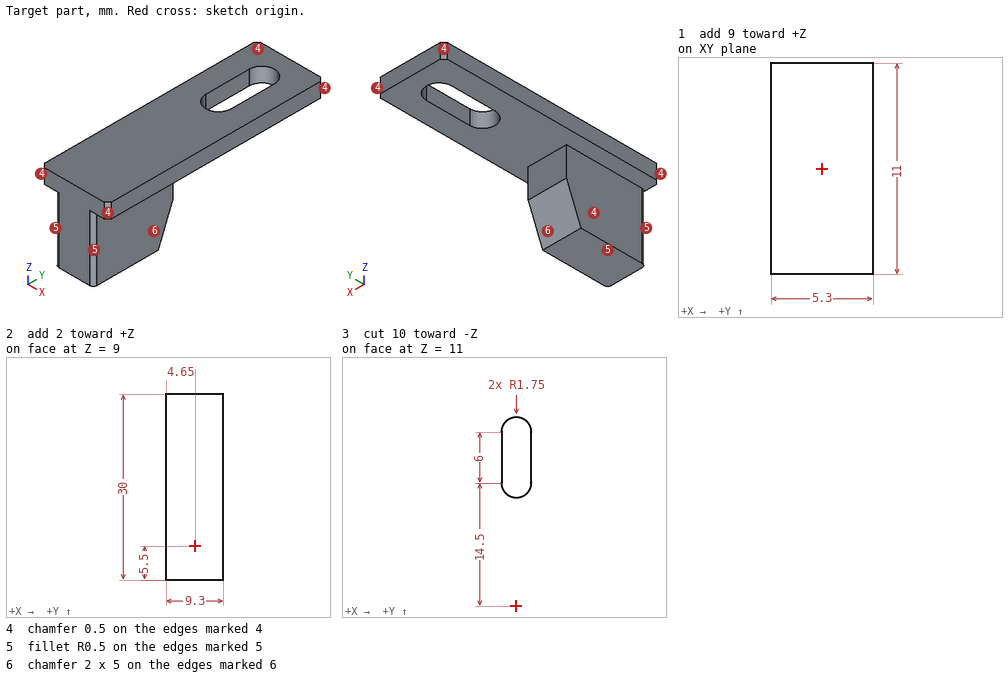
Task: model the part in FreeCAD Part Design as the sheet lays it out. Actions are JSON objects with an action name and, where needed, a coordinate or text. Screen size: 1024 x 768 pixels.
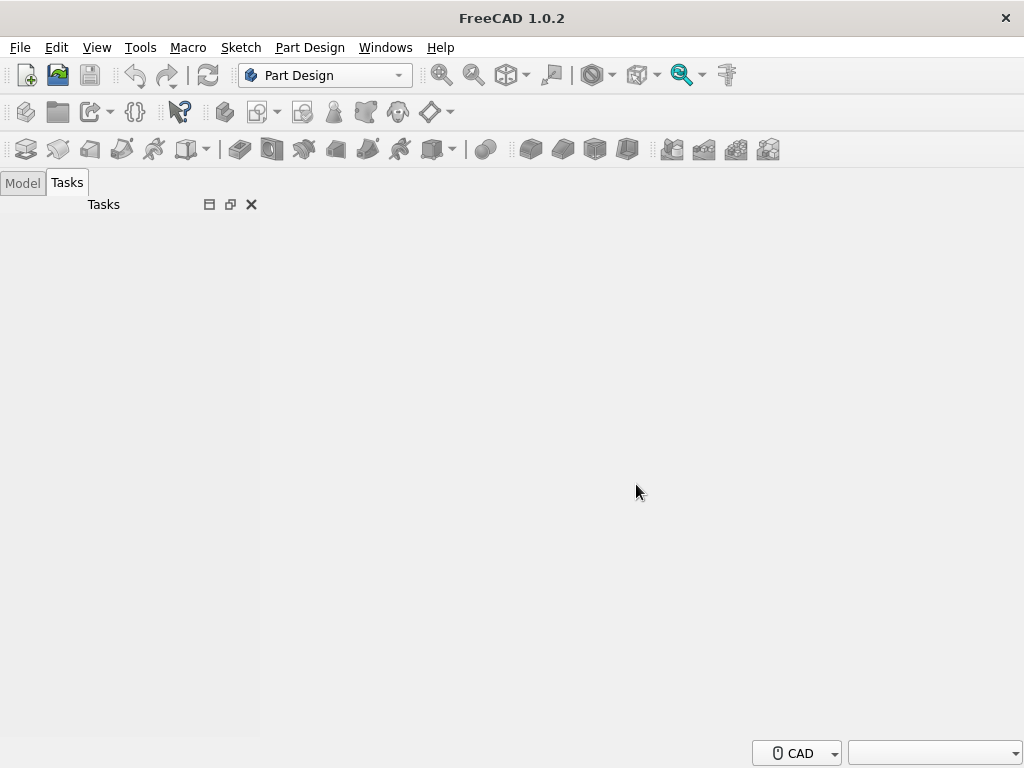
{"action": "left_click", "coordinate": [26, 76]}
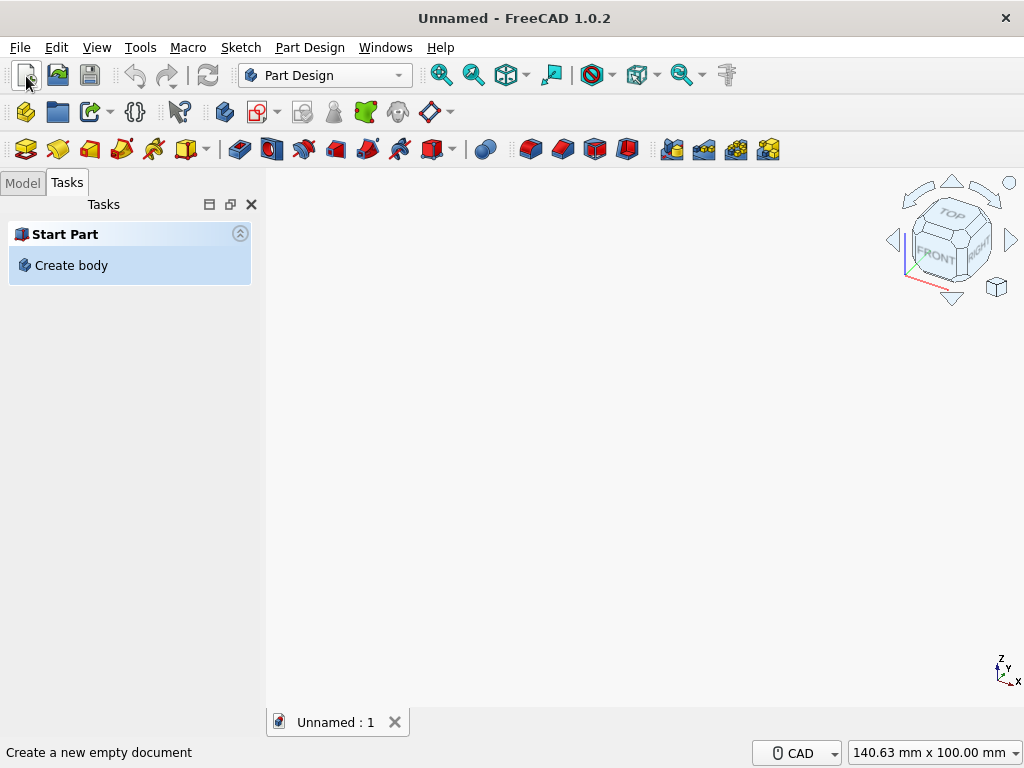
{"action": "left_click", "coordinate": [258, 112]}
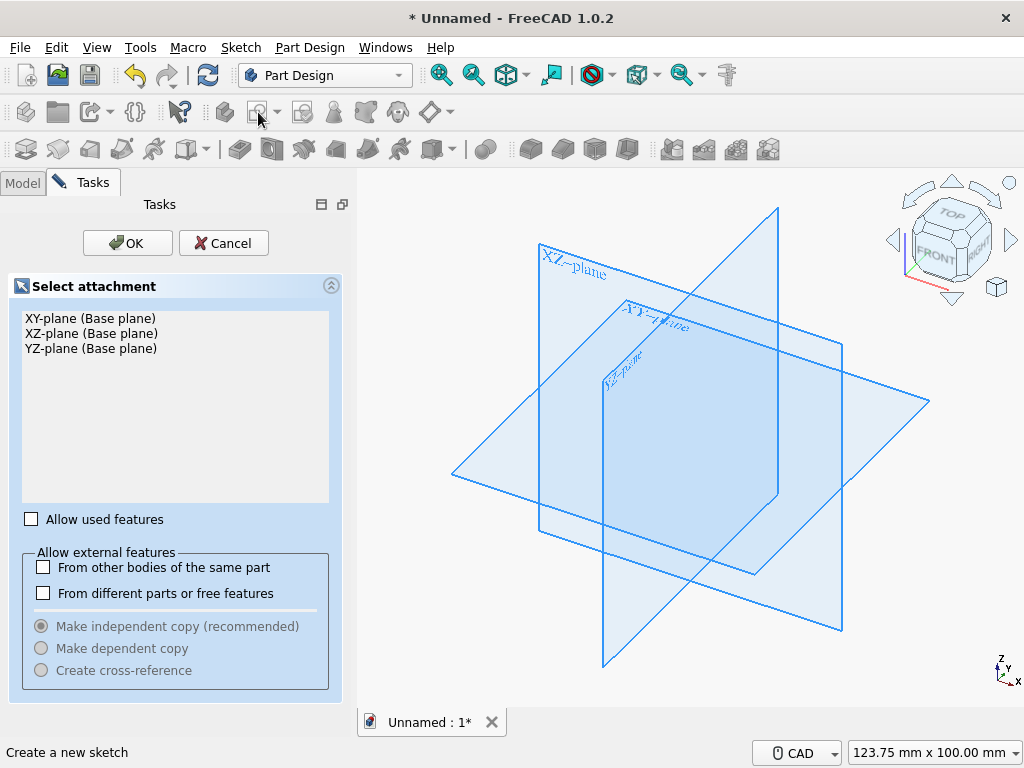
{"action": "left_click", "coordinate": [82, 318]}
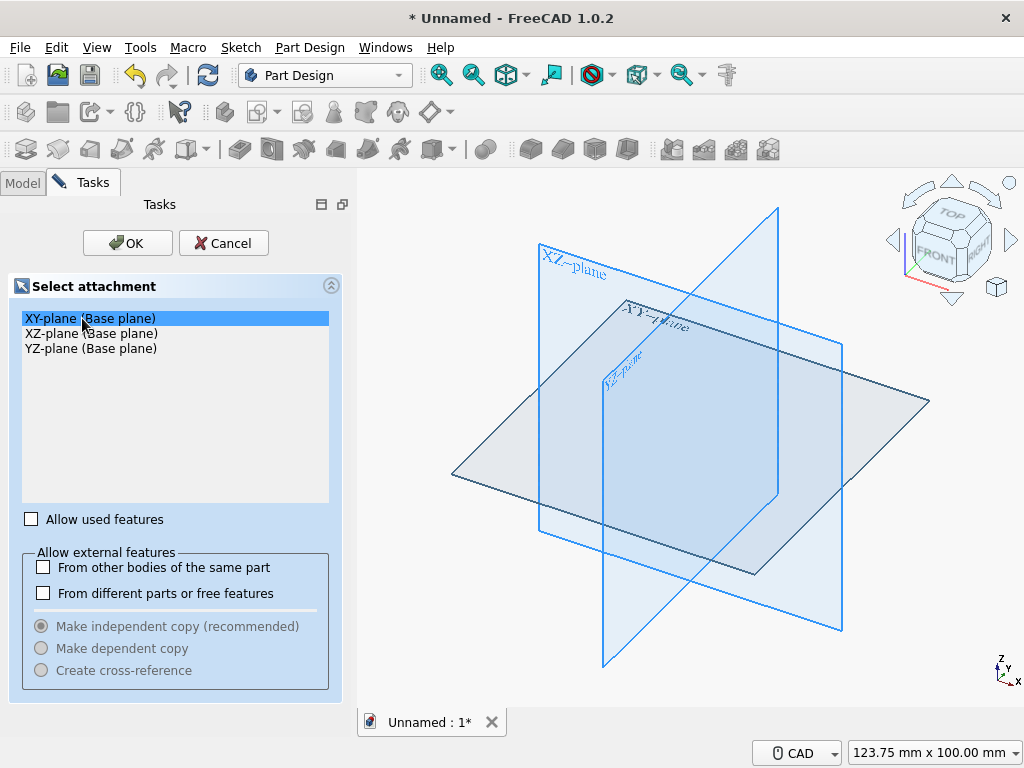
{"action": "left_click", "coordinate": [128, 243]}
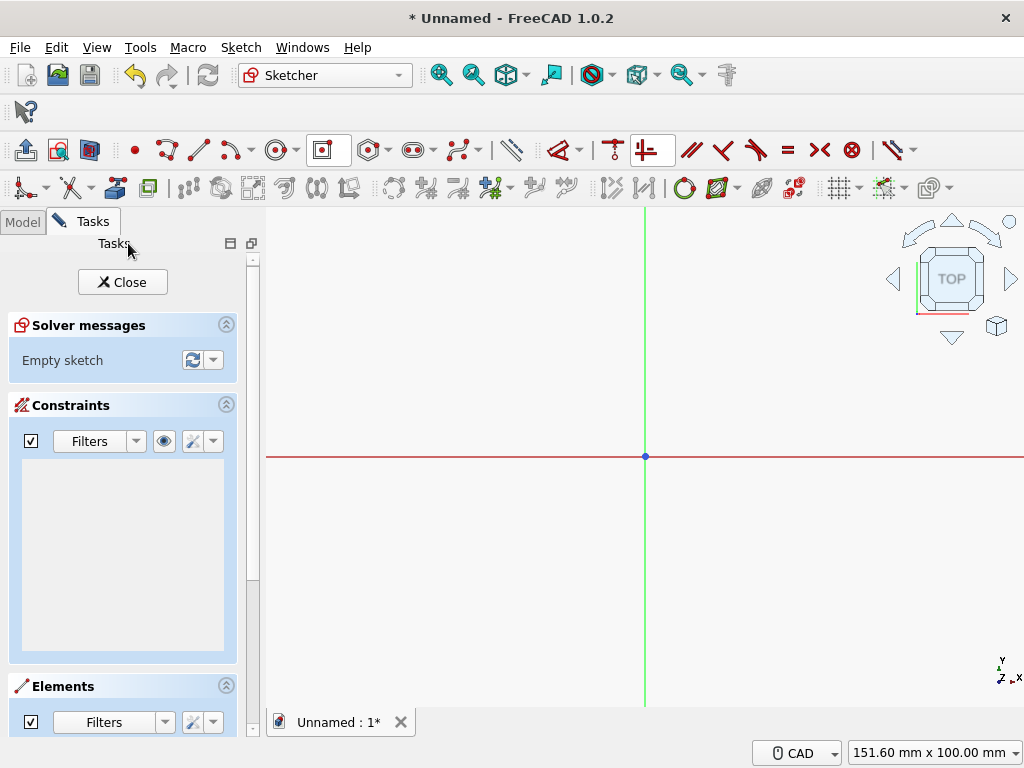
{"action": "scroll", "coordinate": [659, 457], "scroll_direction": "up", "scroll_amount": 9}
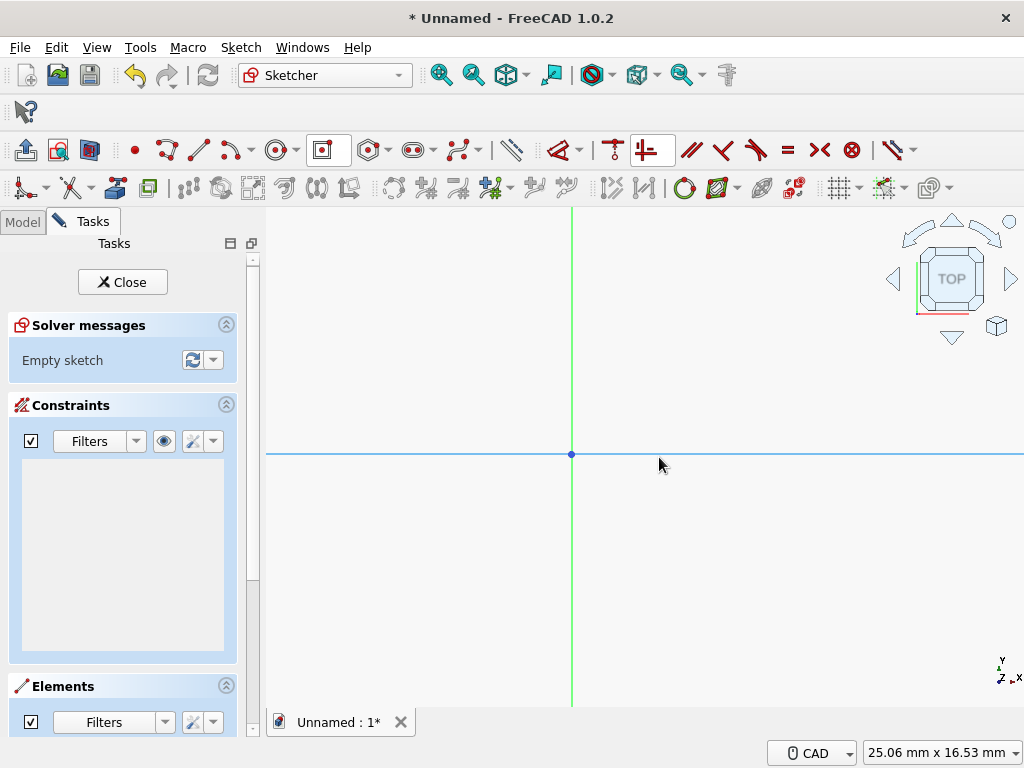
{"action": "left_click", "coordinate": [322, 150]}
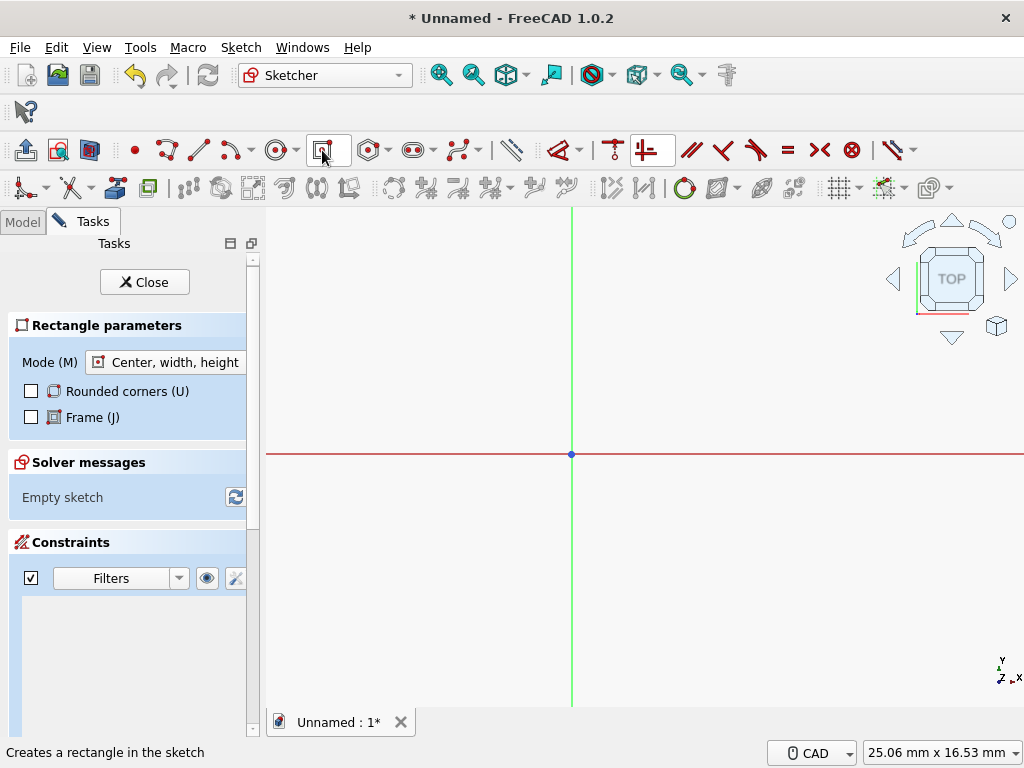
{"action": "left_click", "coordinate": [572, 454]}
{"action": "left_click", "coordinate": [652, 288]}
{"action": "key", "text": "Escape"}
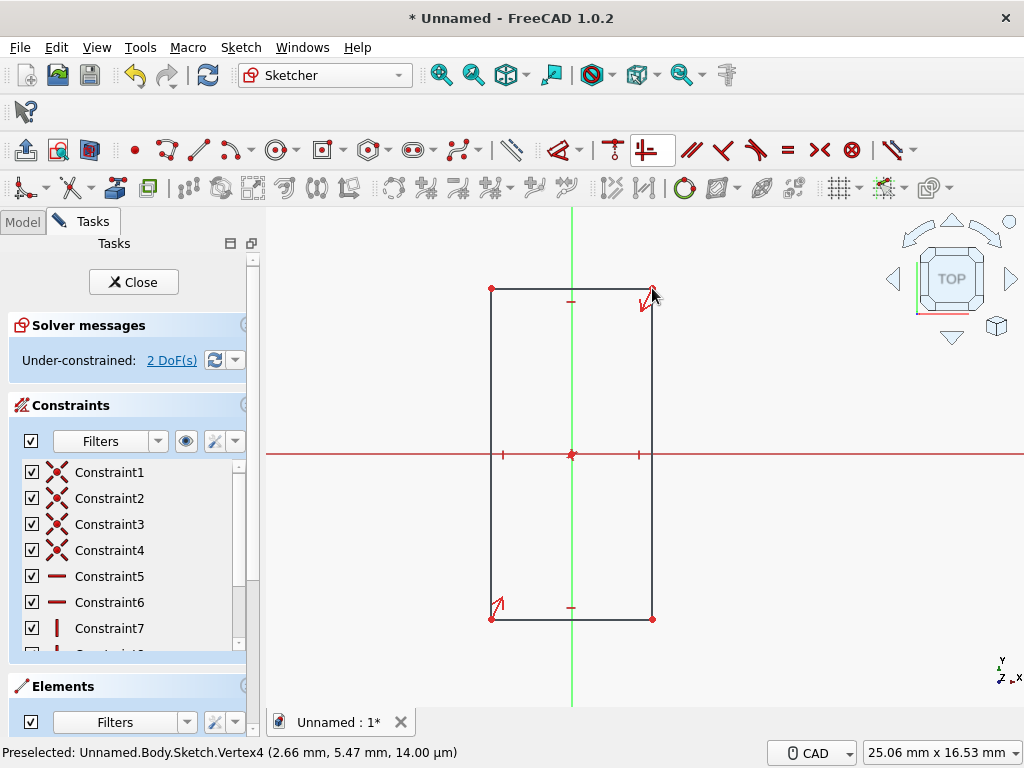
{"action": "left_click", "coordinate": [558, 150]}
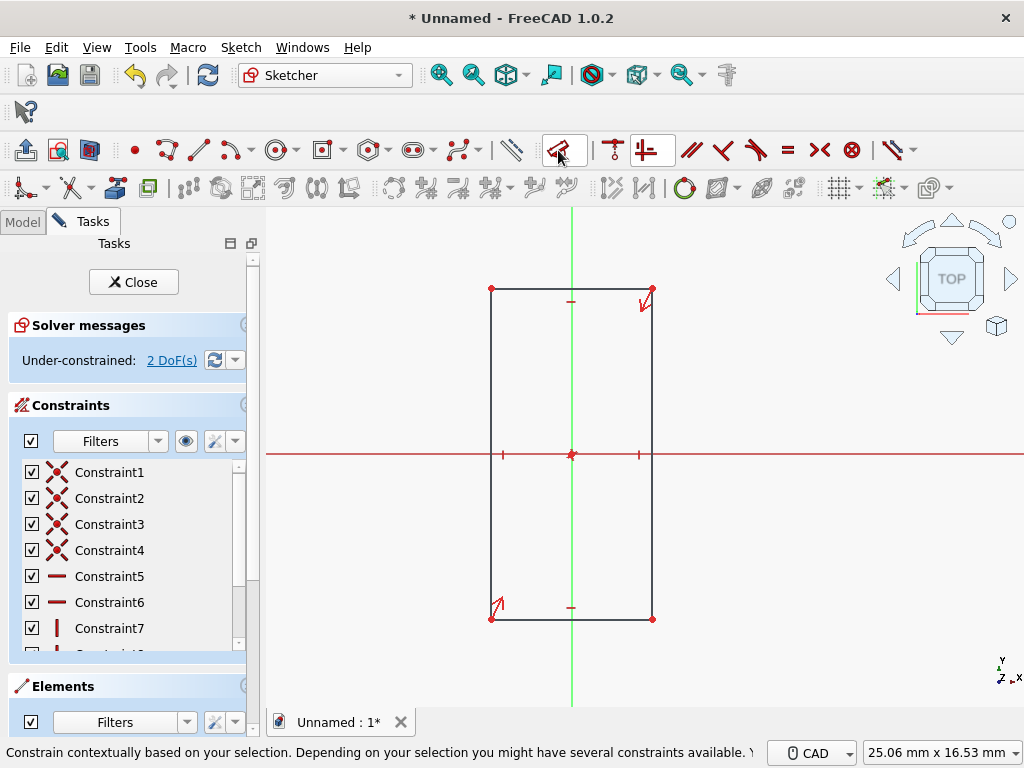
{"action": "left_click", "coordinate": [652, 521]}
{"action": "left_click", "coordinate": [686, 378]}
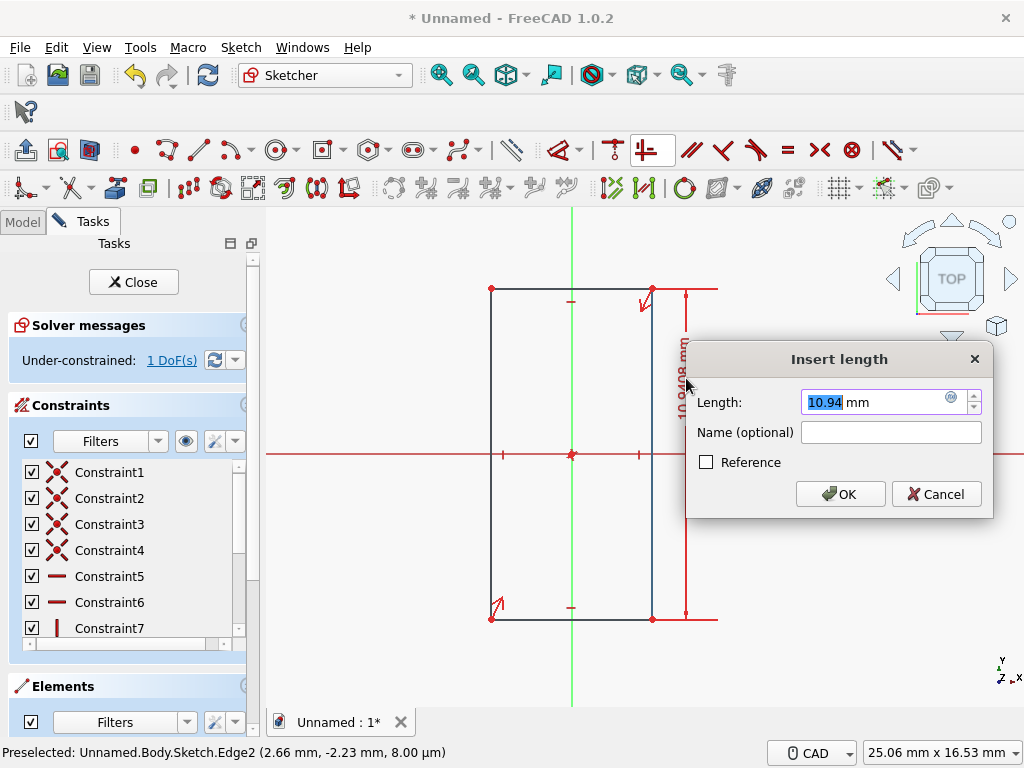
{"action": "type", "text": "11"}
{"action": "key", "text": "Return"}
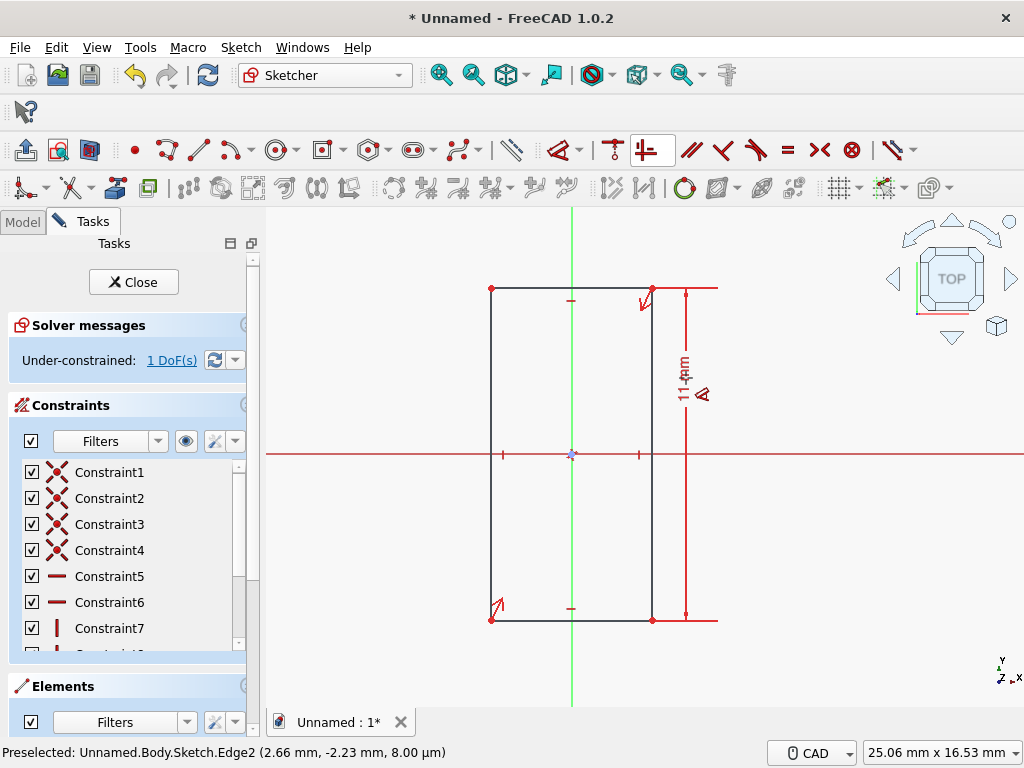
{"action": "left_click", "coordinate": [540, 621]}
{"action": "left_click", "coordinate": [535, 655]}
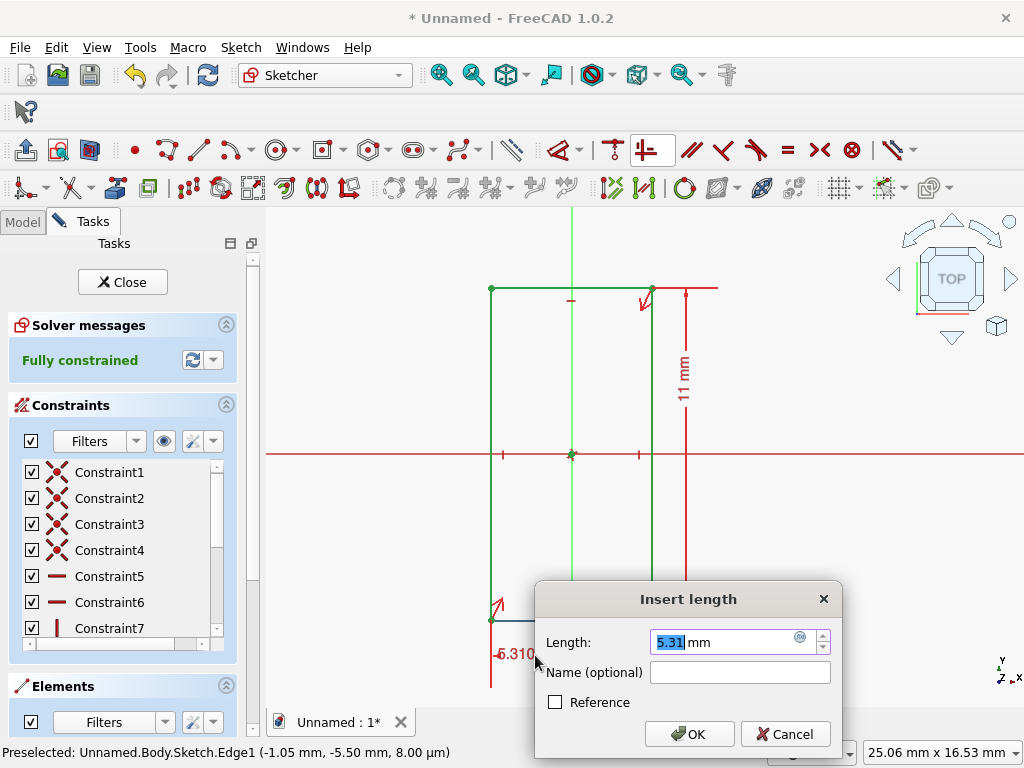
{"action": "type", "text": "5.3"}
{"action": "key", "text": "Return"}
{"action": "key", "text": "Escape"}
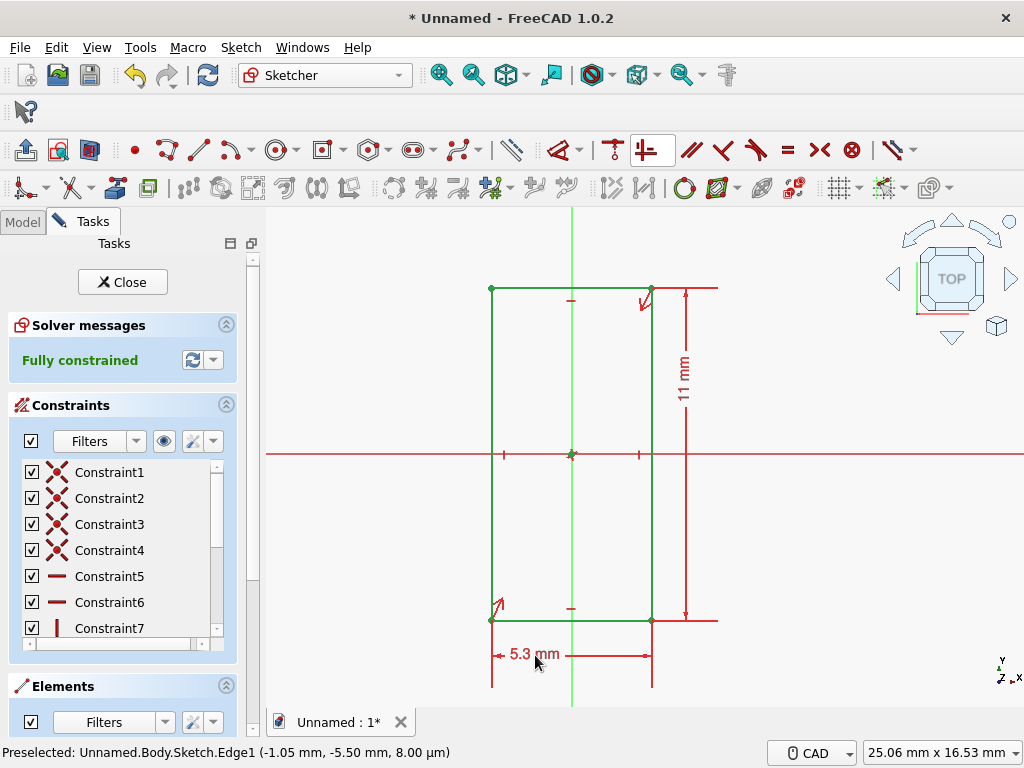
{"action": "left_click", "coordinate": [123, 282]}